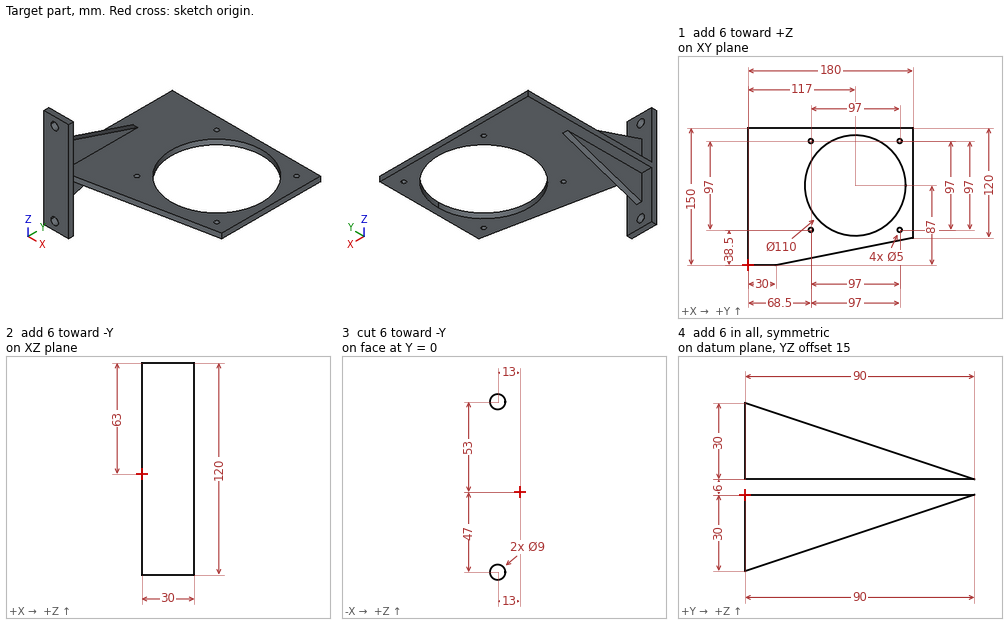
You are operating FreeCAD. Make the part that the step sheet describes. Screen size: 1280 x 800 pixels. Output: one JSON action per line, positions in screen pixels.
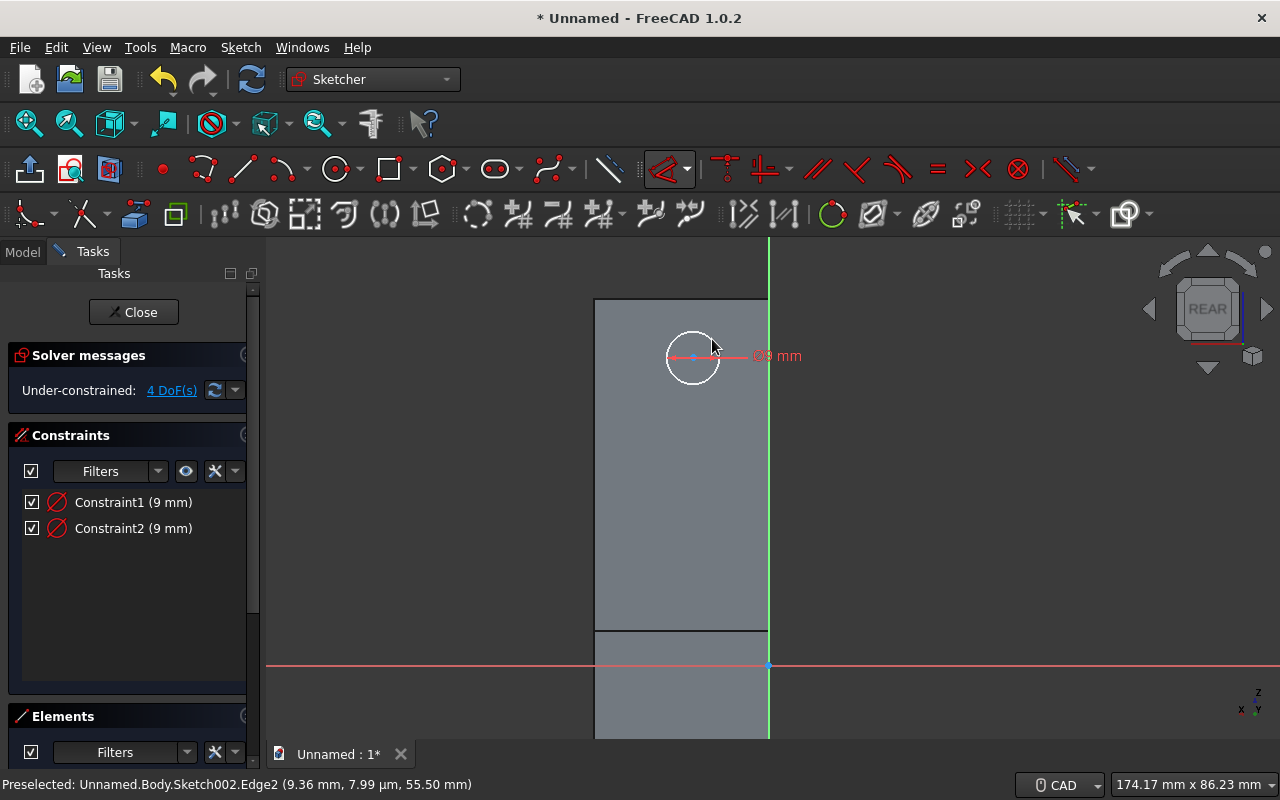
{"action": "scroll", "coordinate": [694, 357], "scroll_direction": "down", "scroll_amount": 4}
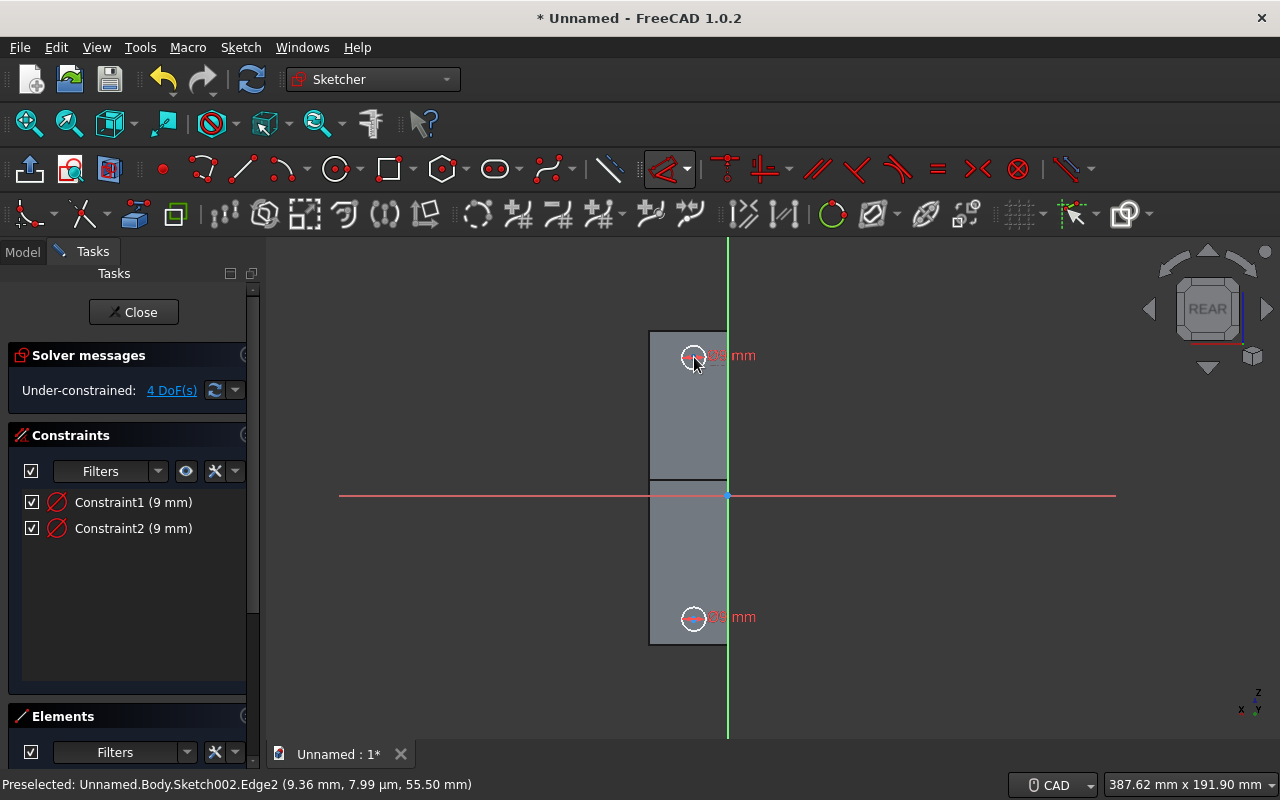
{"action": "left_click", "coordinate": [694, 619]}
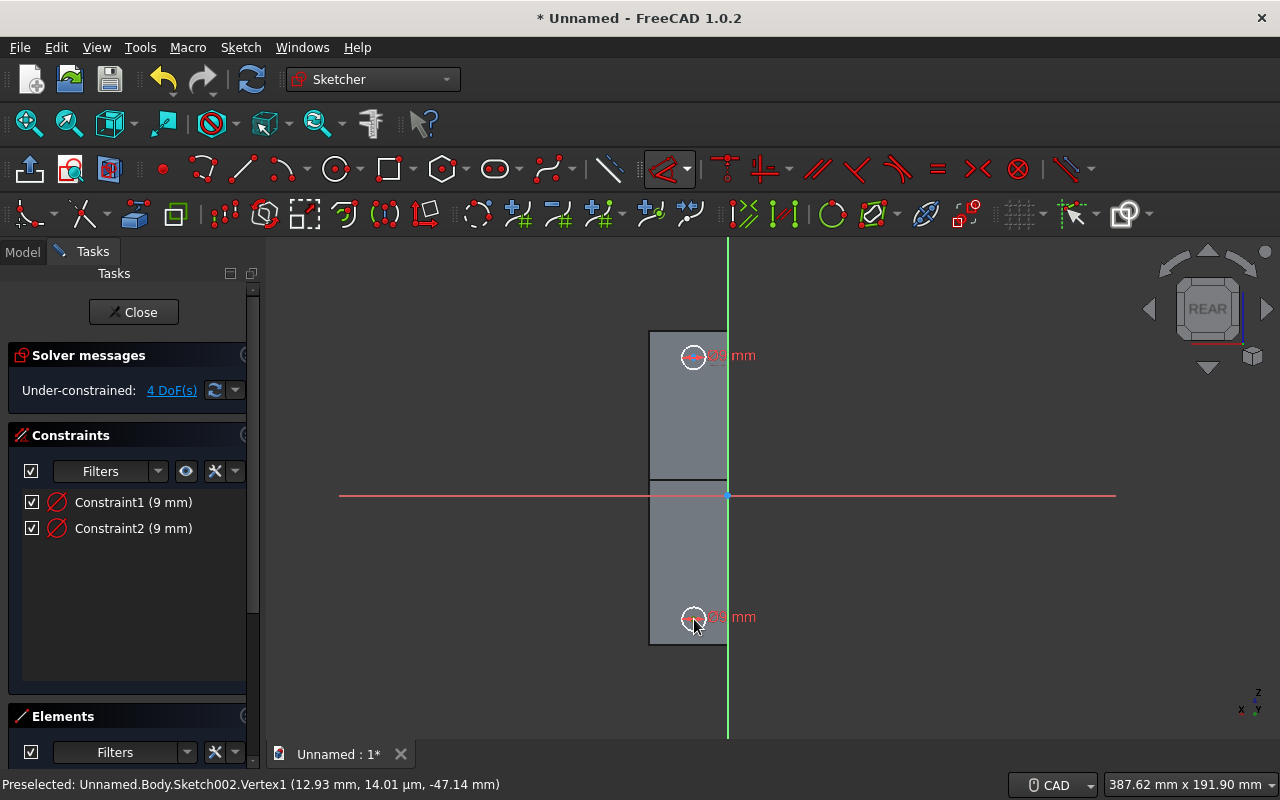
{"action": "key", "text": "l"}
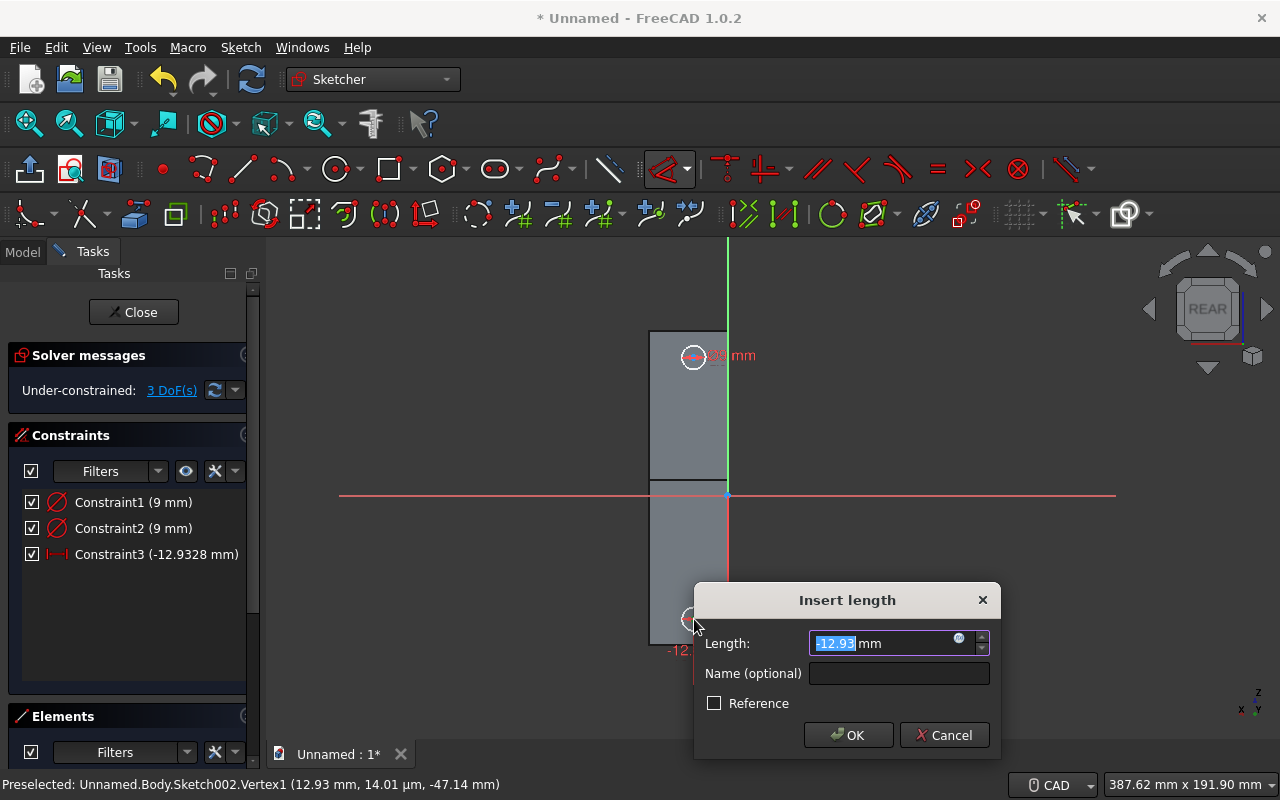
{"action": "type", "text": "-13"}
{"action": "key", "text": "Return"}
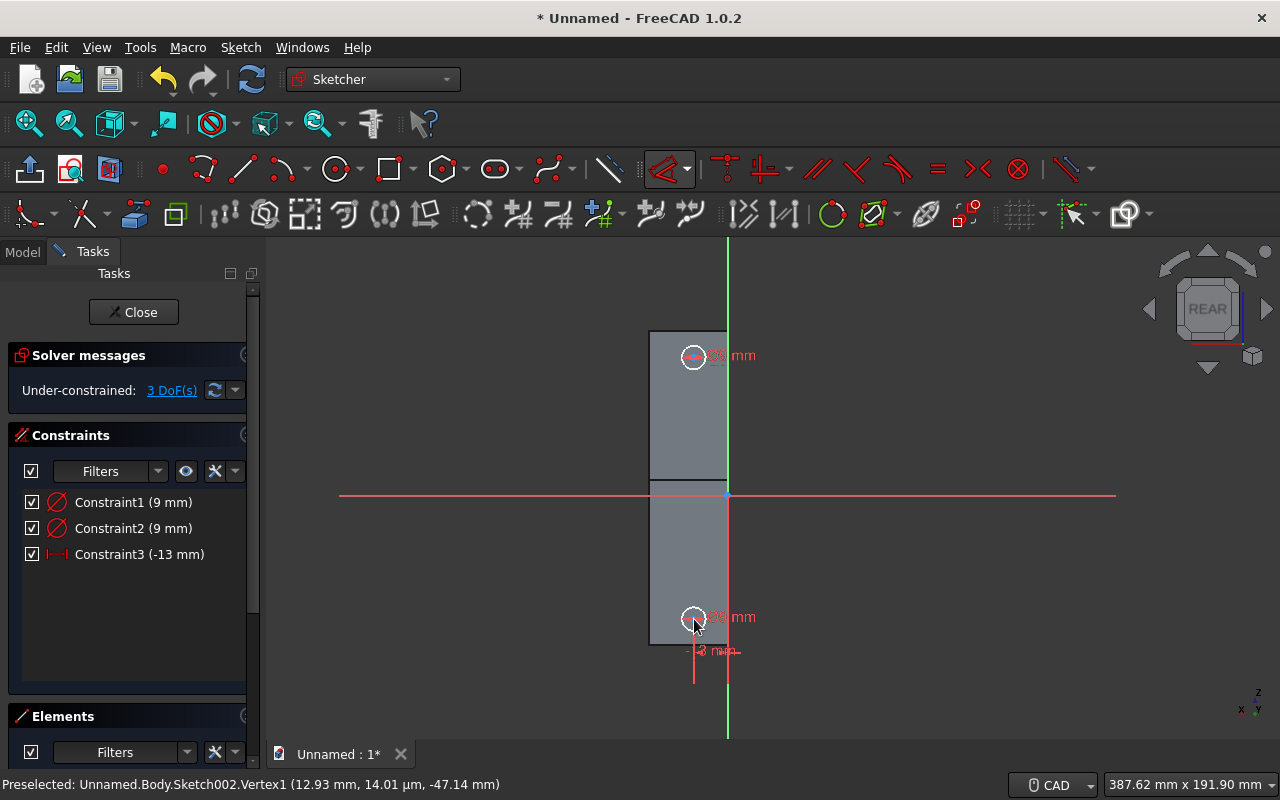
{"action": "left_click", "coordinate": [694, 619]}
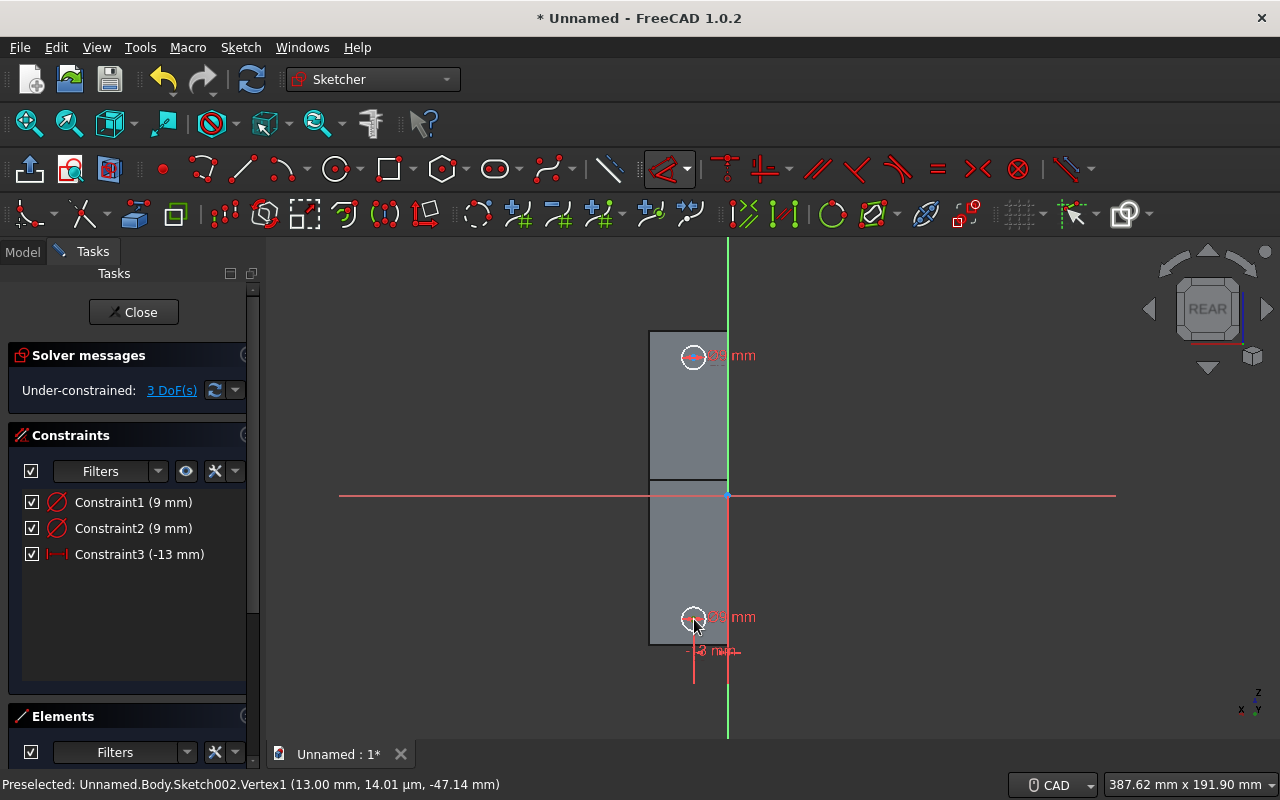
{"action": "key", "text": "i"}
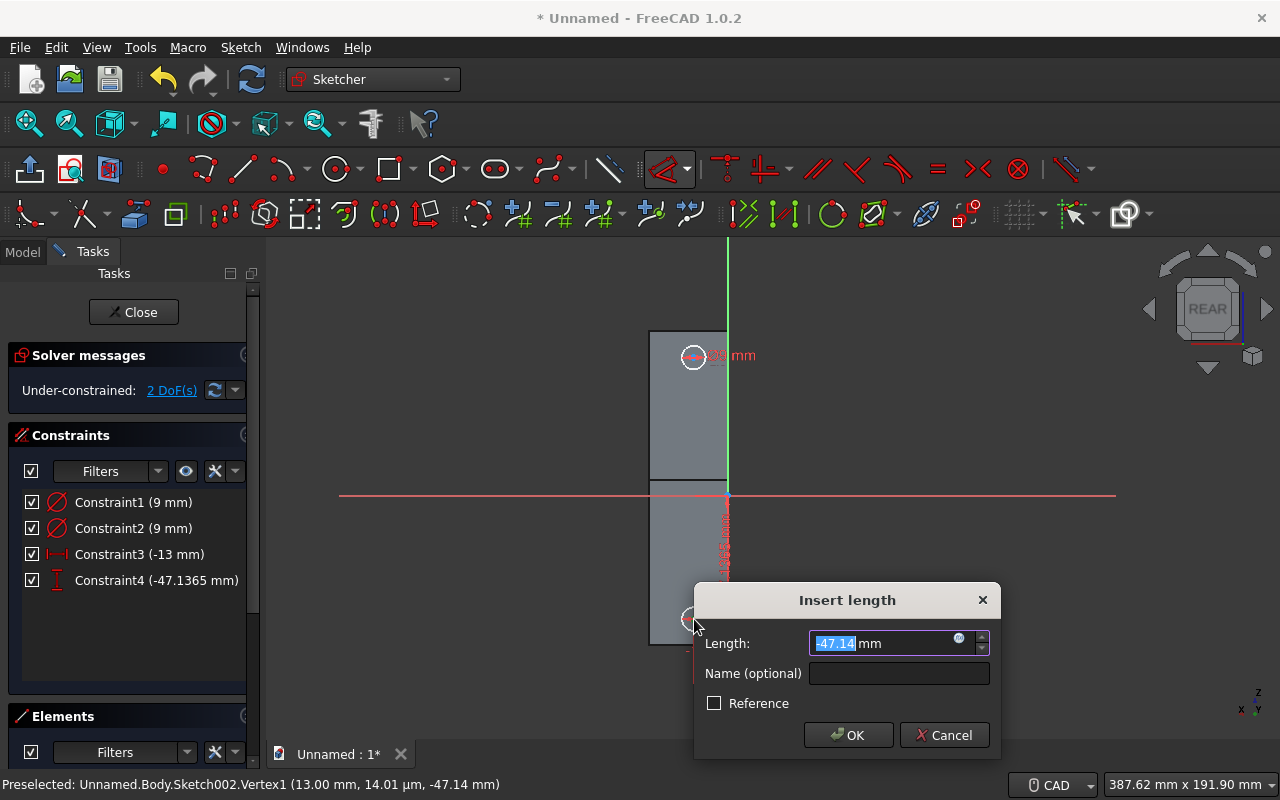
{"action": "type", "text": "-47"}
{"action": "key", "text": "Return"}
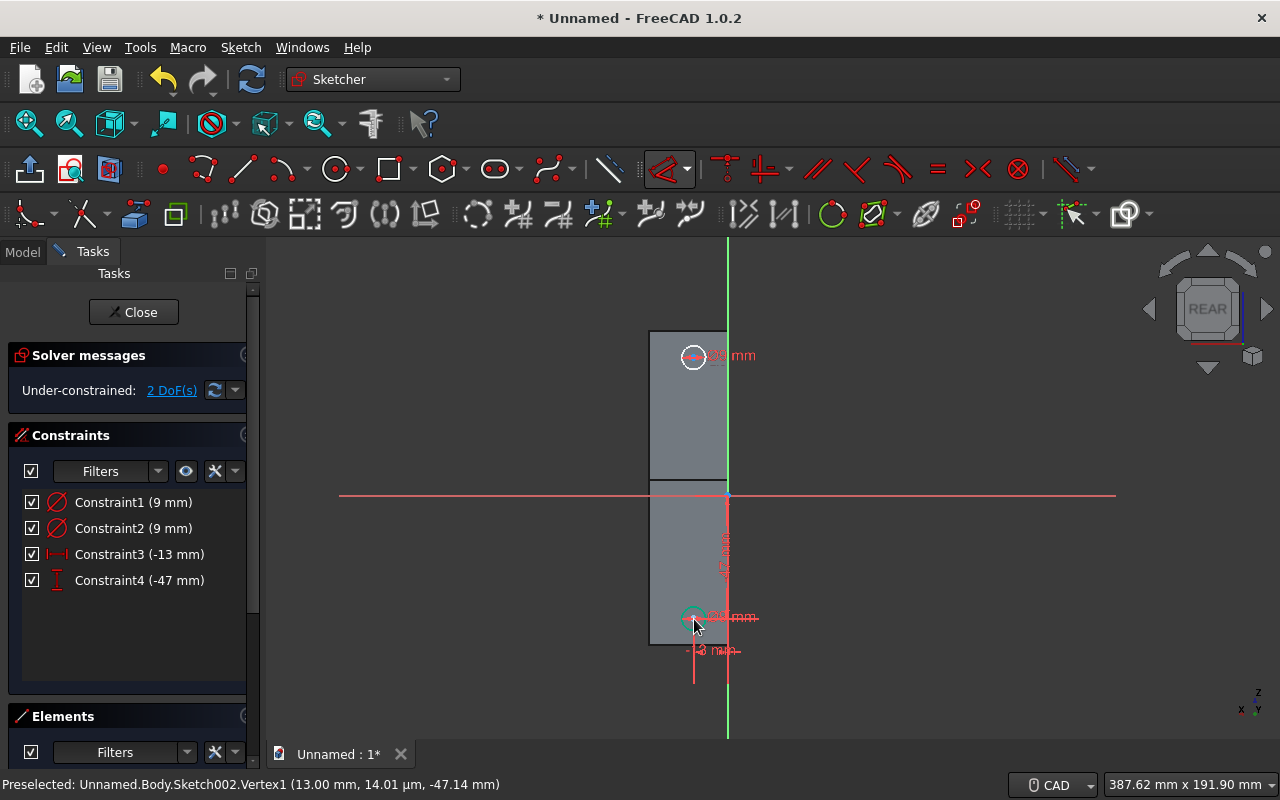
{"action": "left_click", "coordinate": [694, 358]}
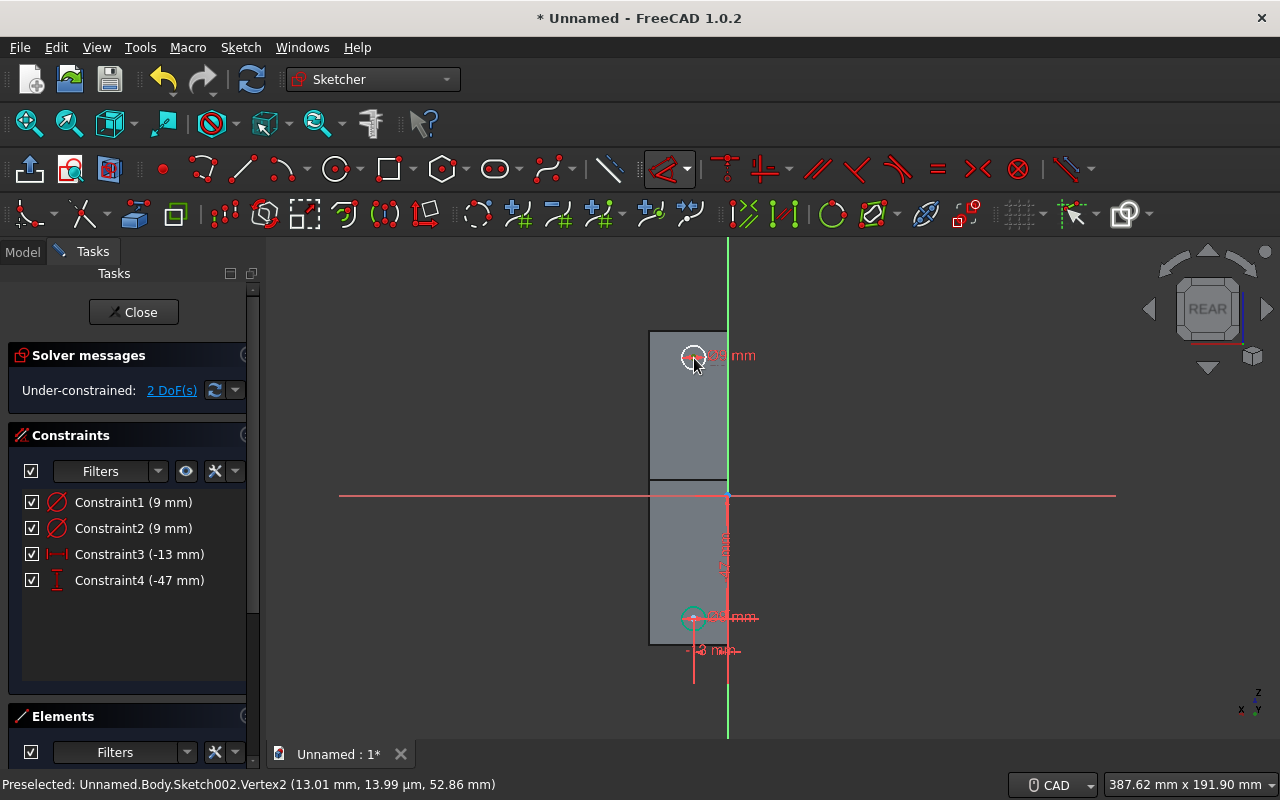
{"action": "key", "text": "l"}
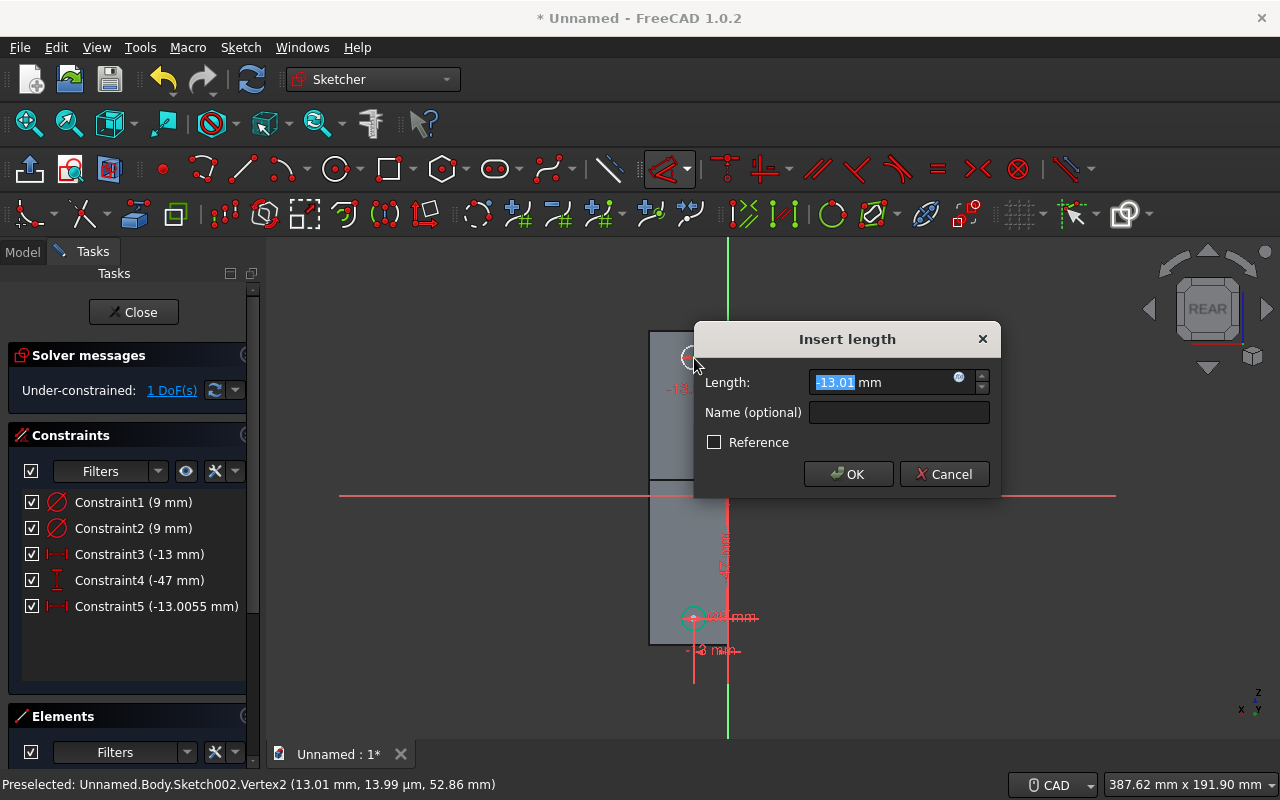
{"action": "type", "text": "-13"}
{"action": "key", "text": "Return"}